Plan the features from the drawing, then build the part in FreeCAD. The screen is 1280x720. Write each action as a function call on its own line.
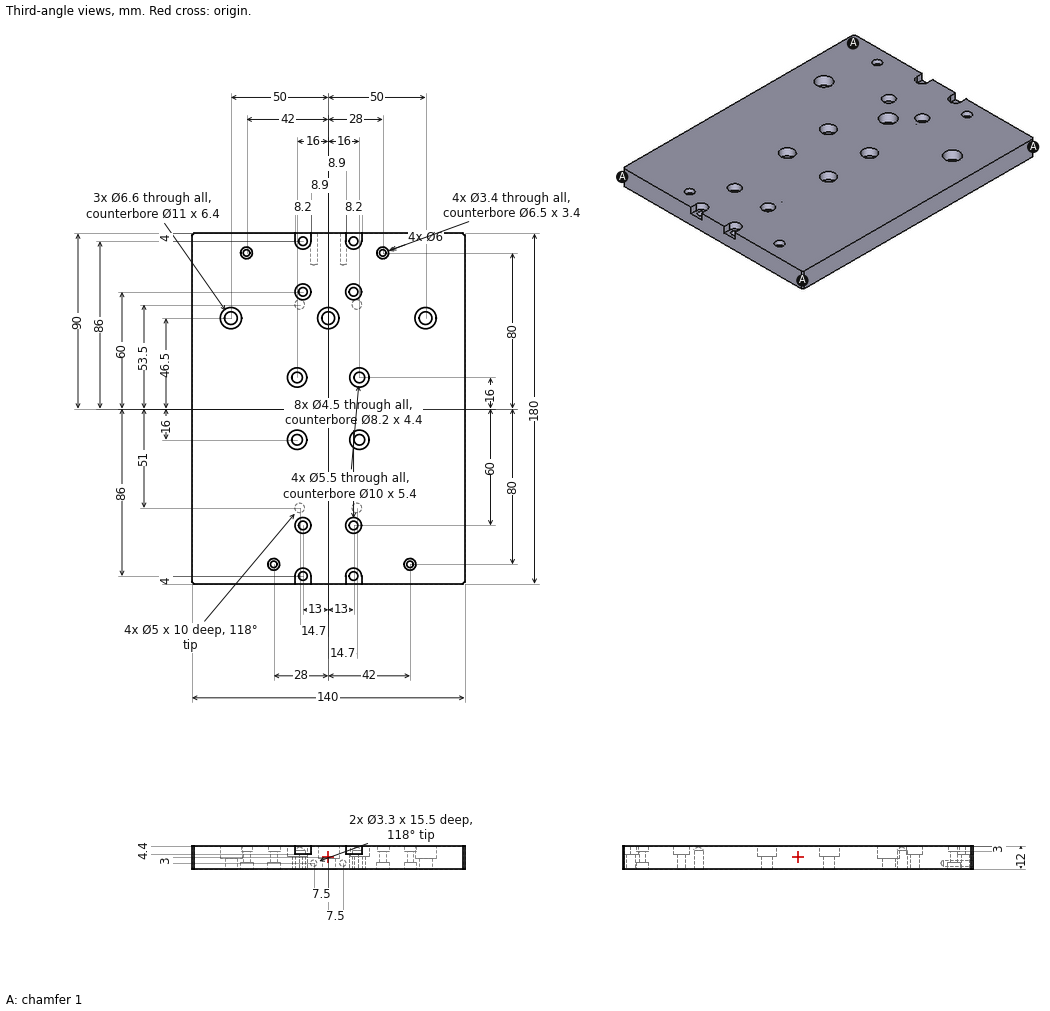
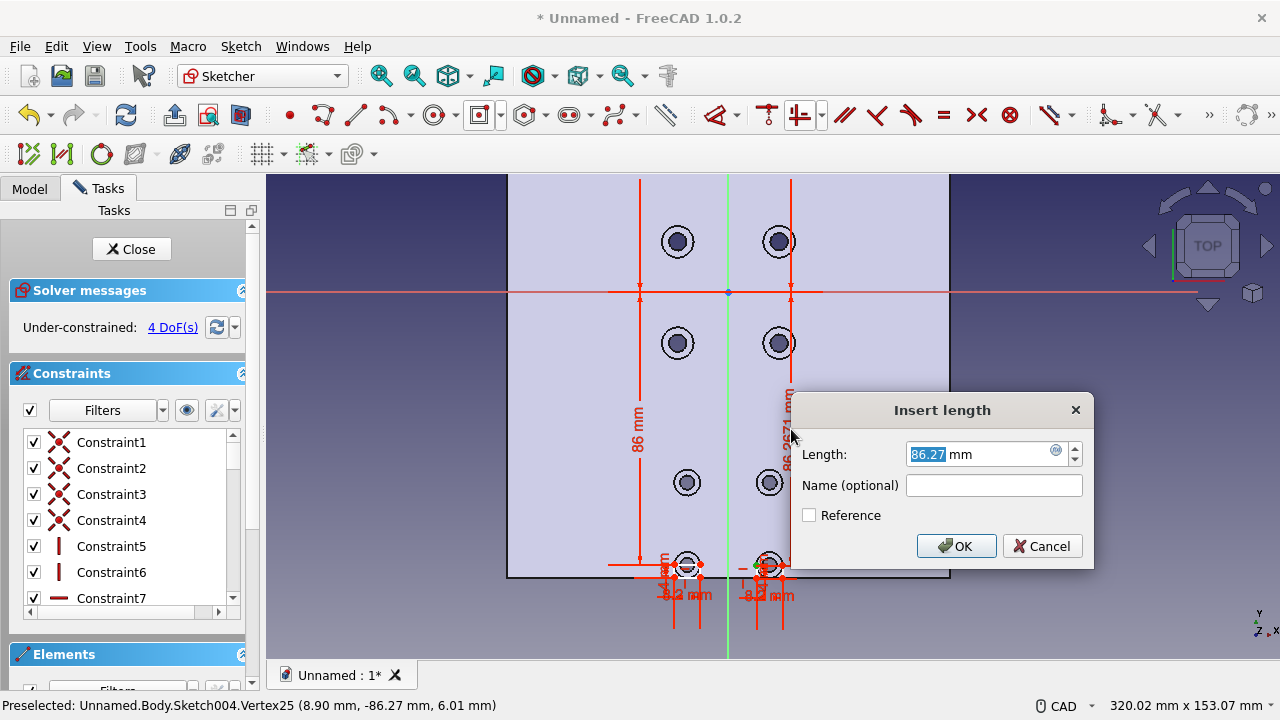
text(86)
key(Return)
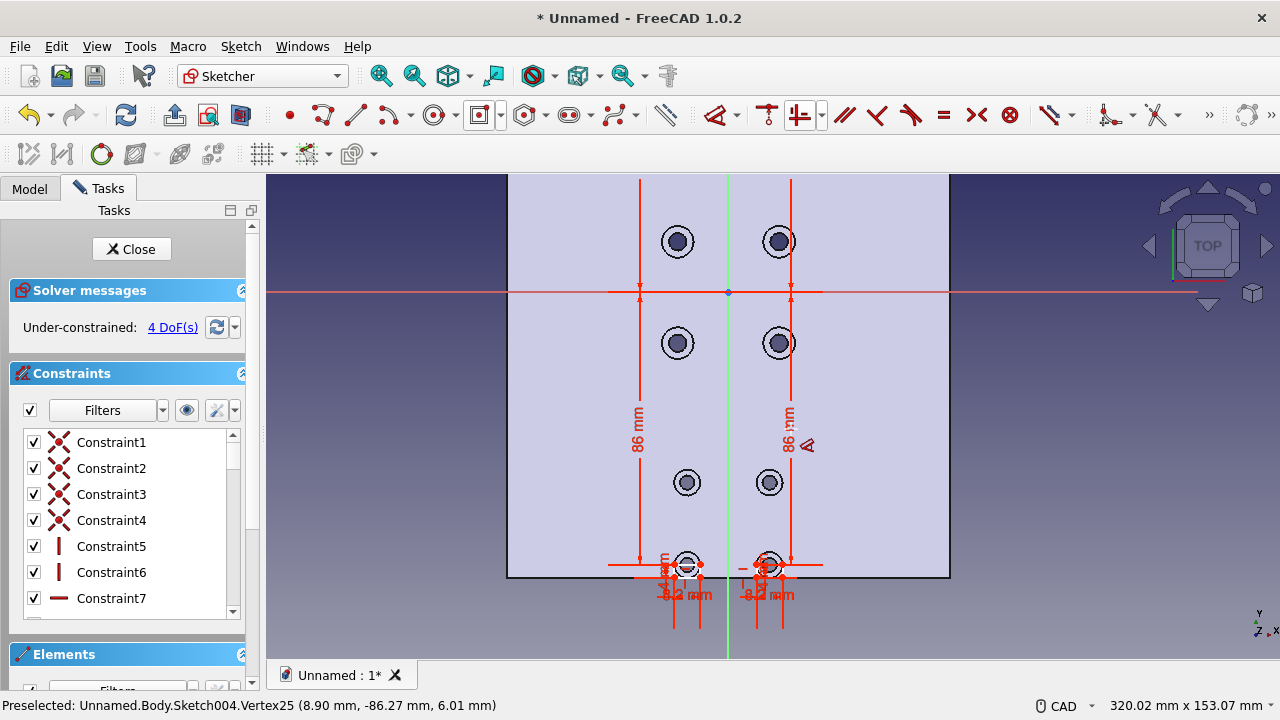
scroll(675, 567, down, 3)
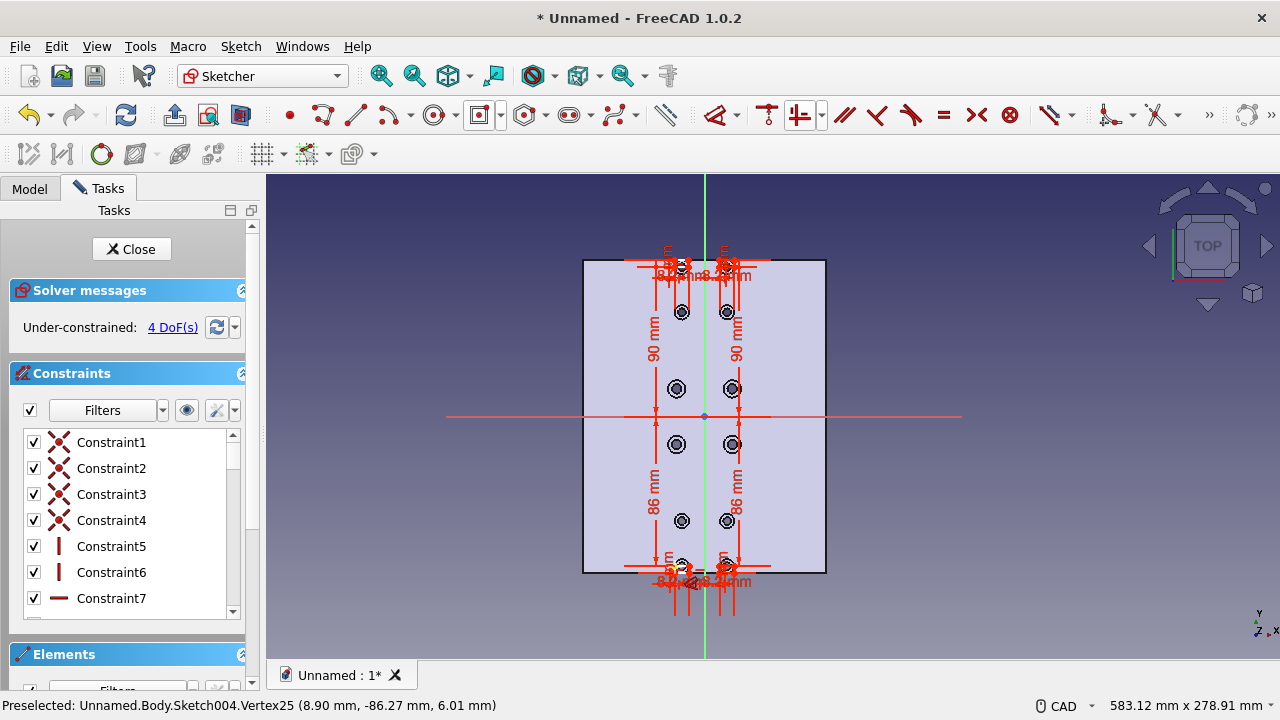
scroll(689, 267, up, 5)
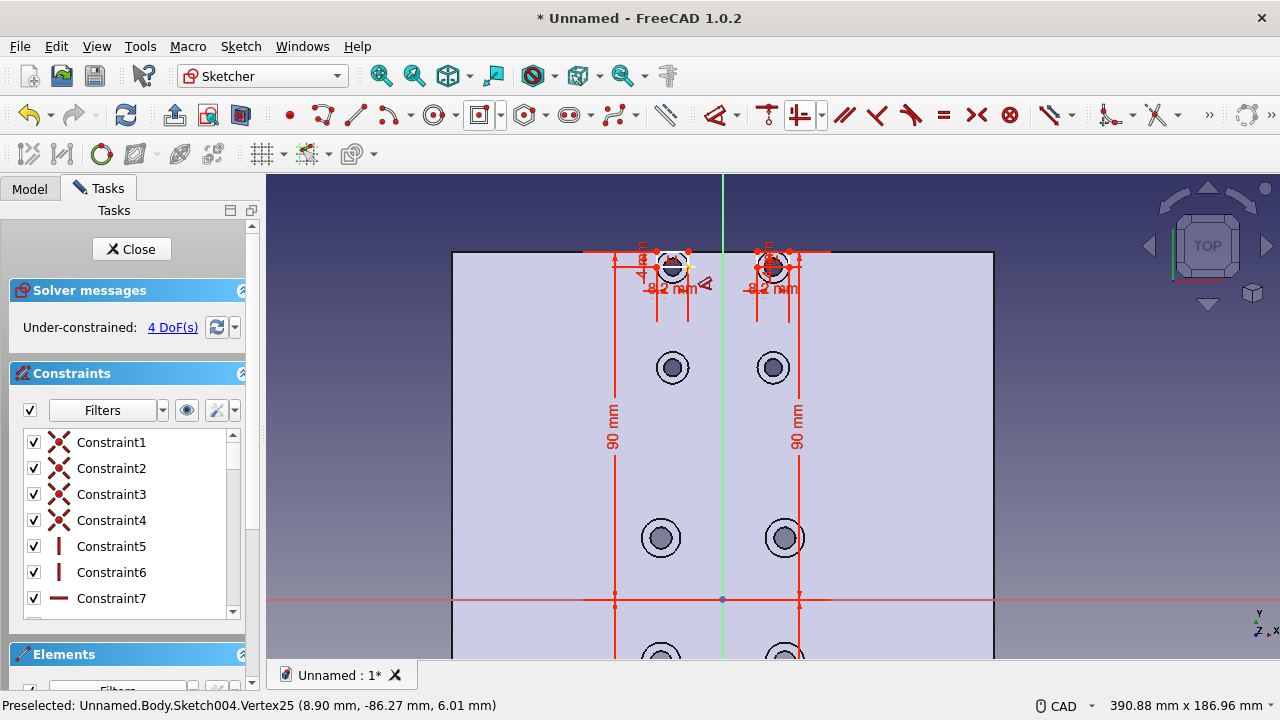
click(688, 267)
click(709, 233)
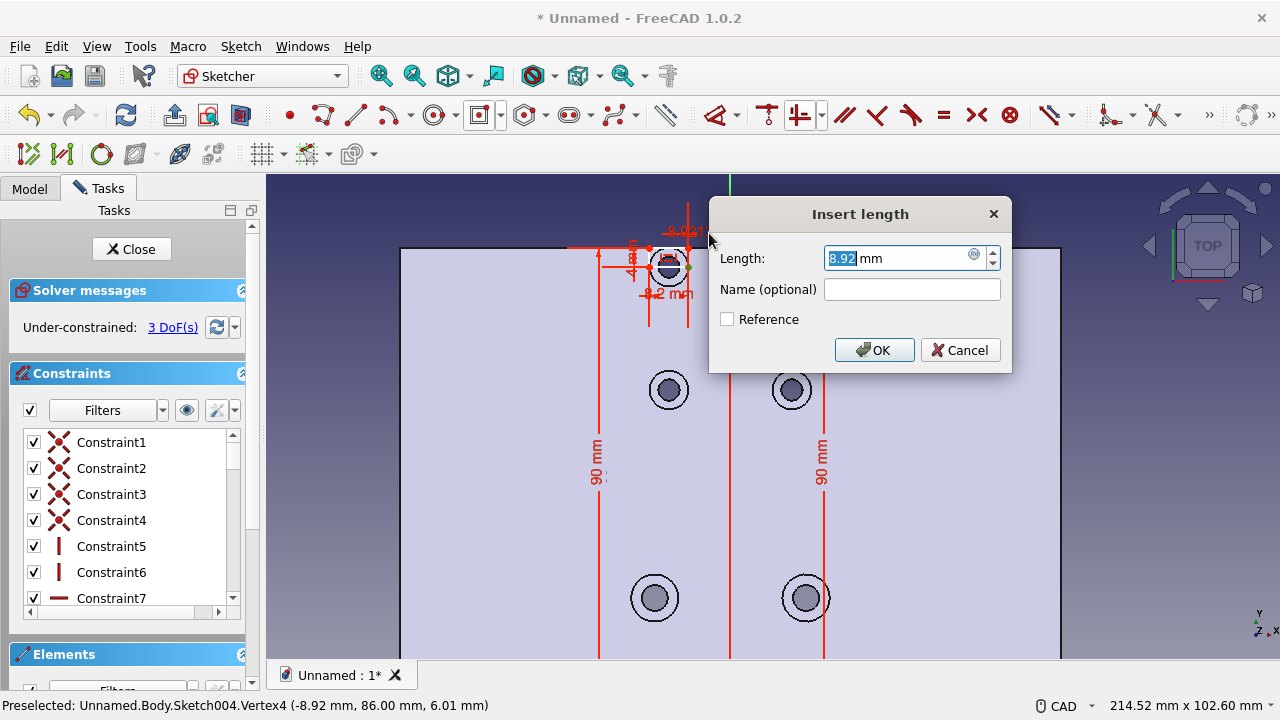
text(8.9)
key(Return)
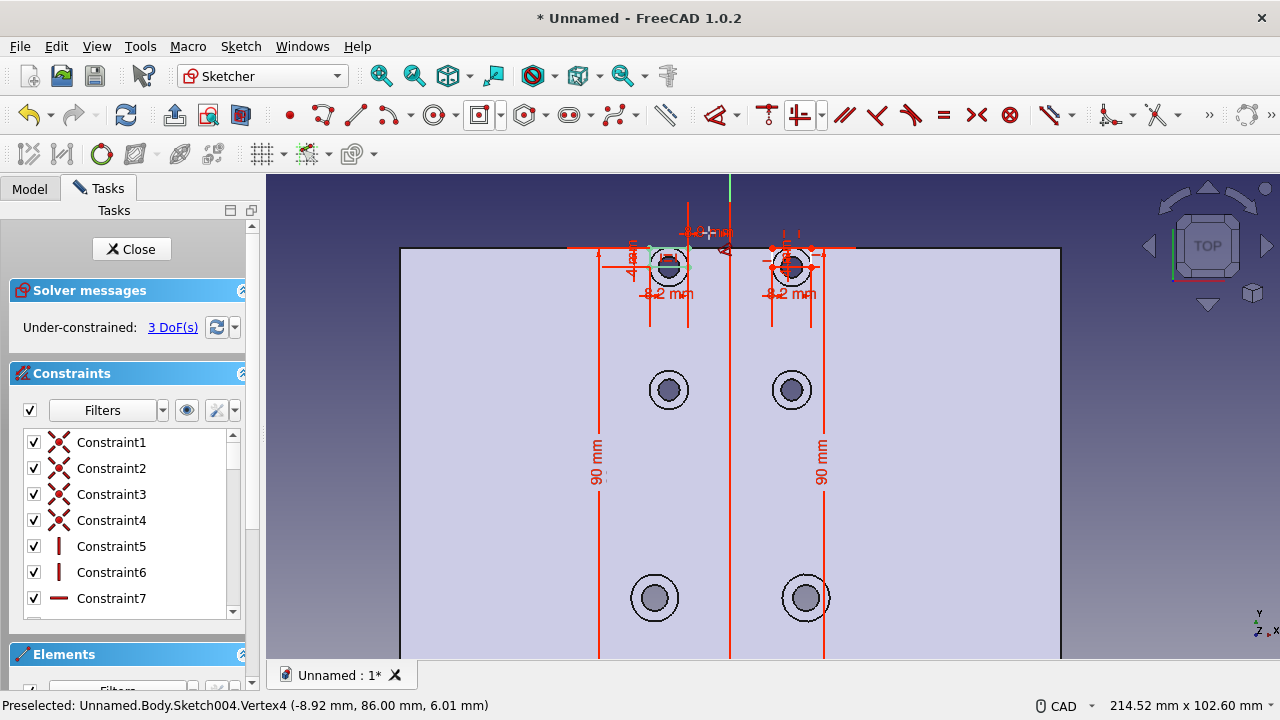
click(772, 248)
click(751, 214)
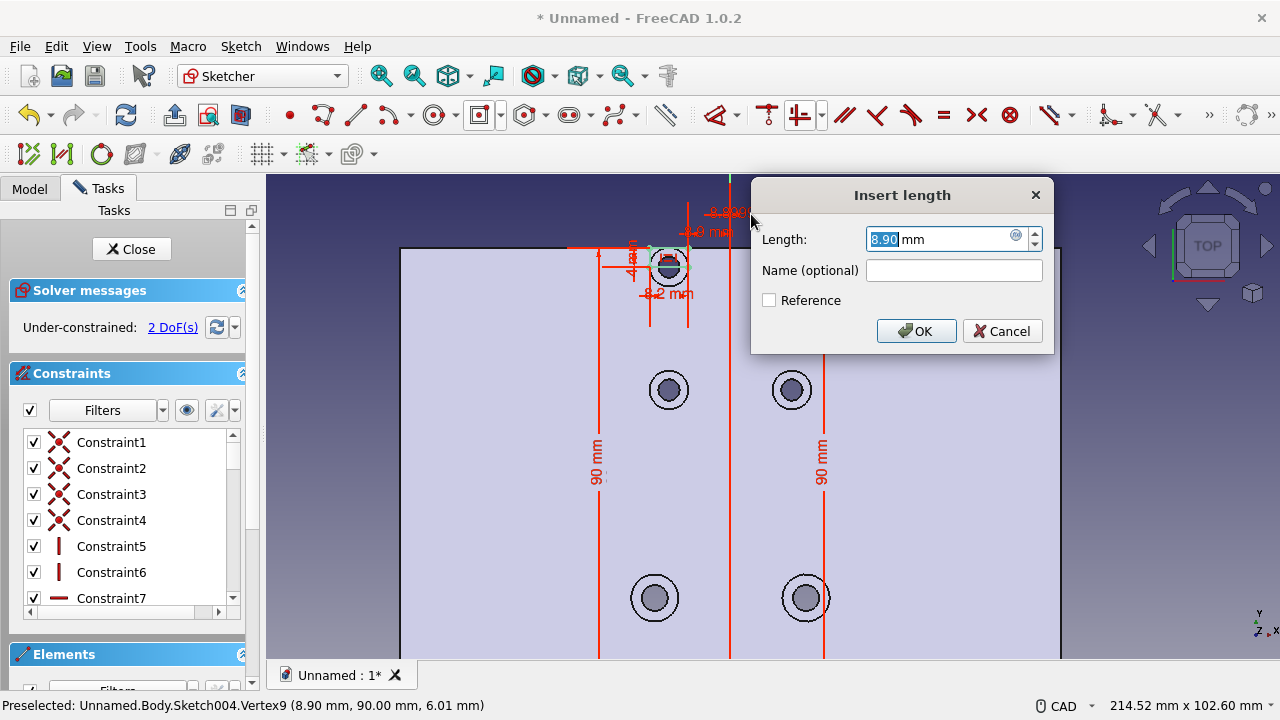
text(8.9)
key(Return)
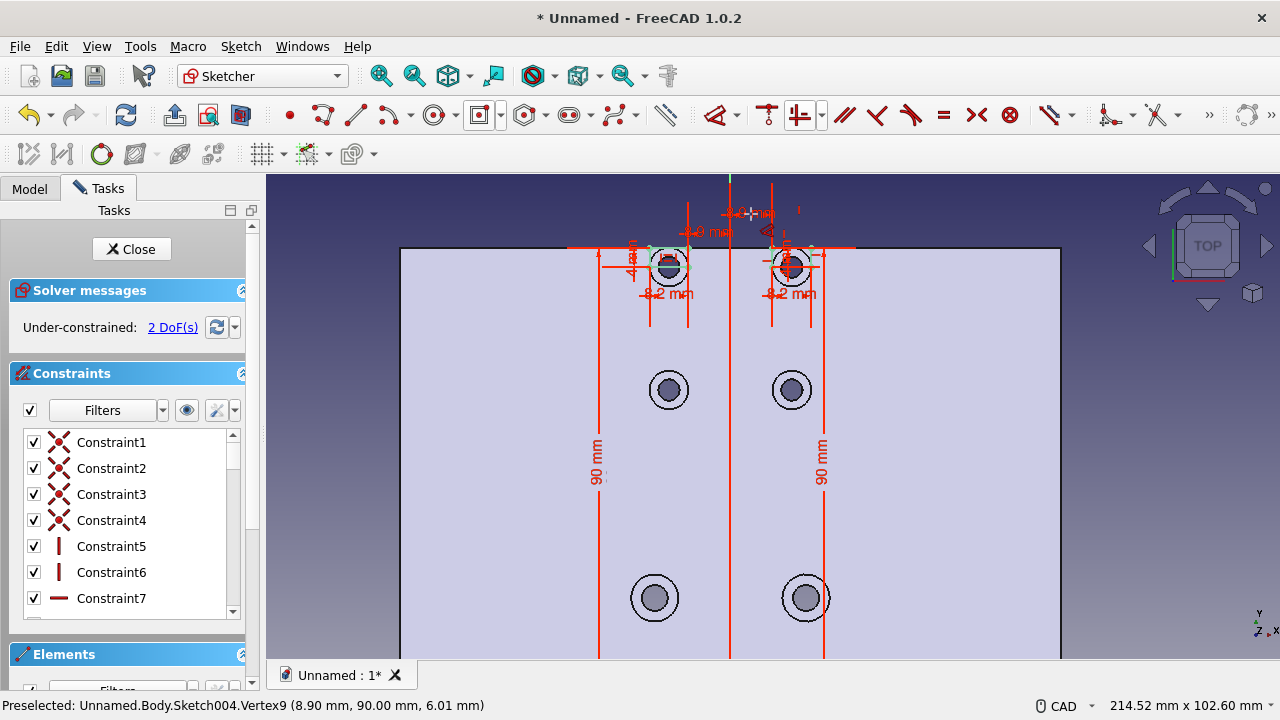
scroll(689, 267, down, 5)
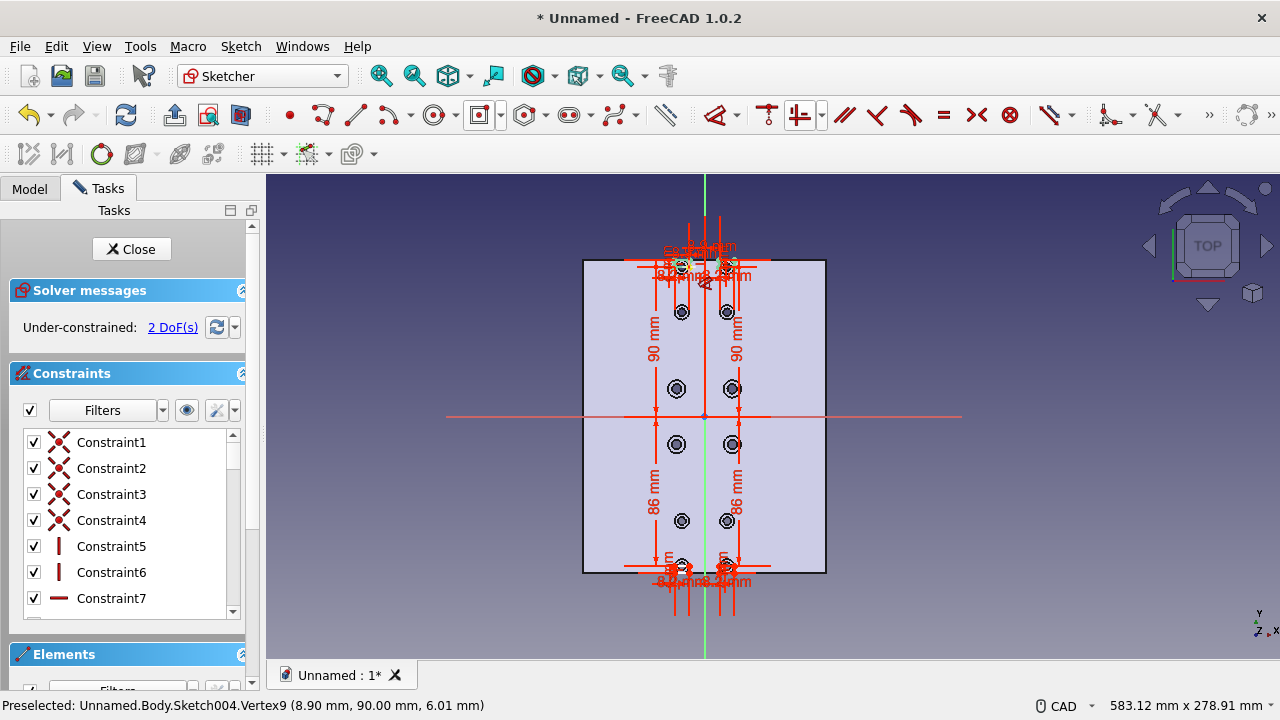
scroll(689, 573, up, 5)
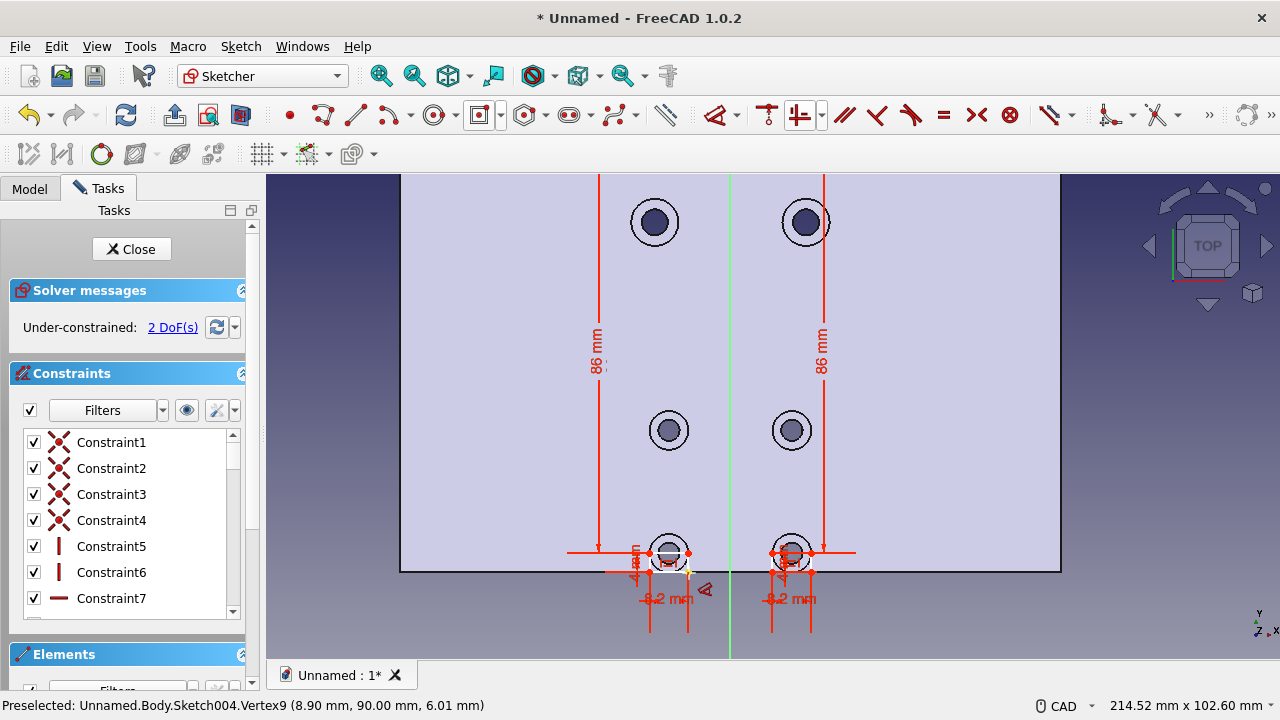
click(688, 572)
click(709, 630)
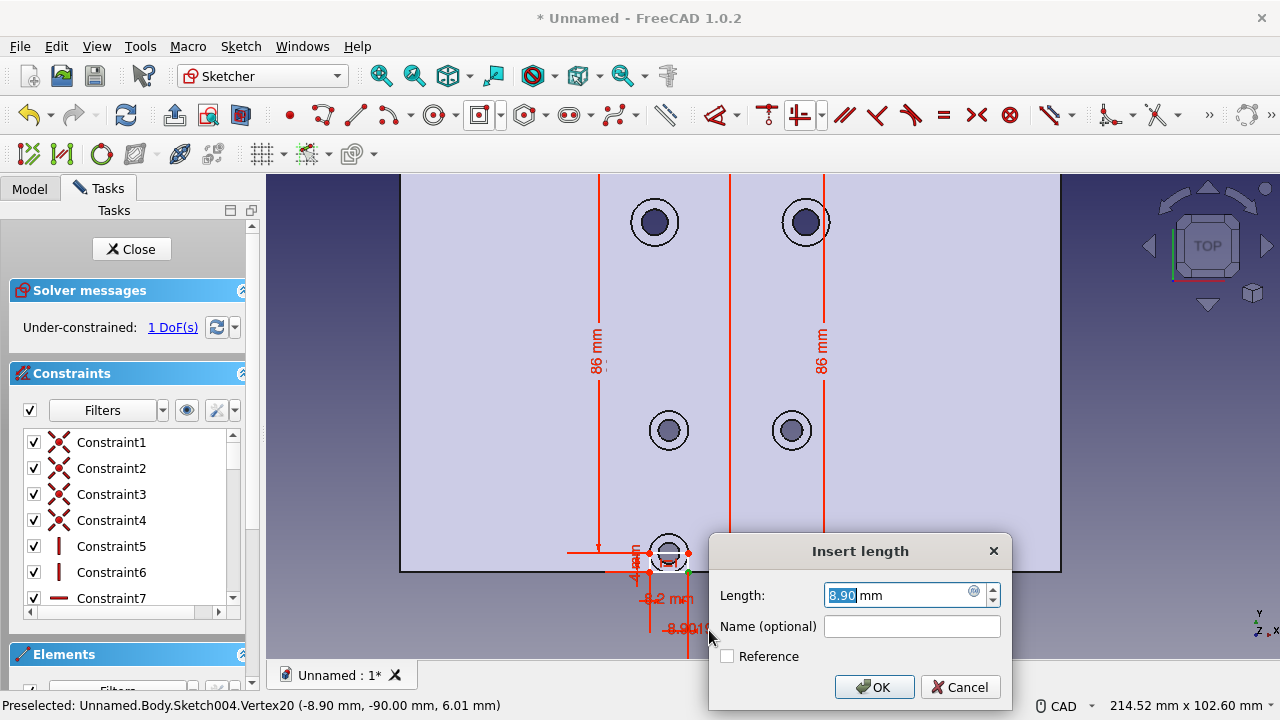
text(8.9)
key(Return)